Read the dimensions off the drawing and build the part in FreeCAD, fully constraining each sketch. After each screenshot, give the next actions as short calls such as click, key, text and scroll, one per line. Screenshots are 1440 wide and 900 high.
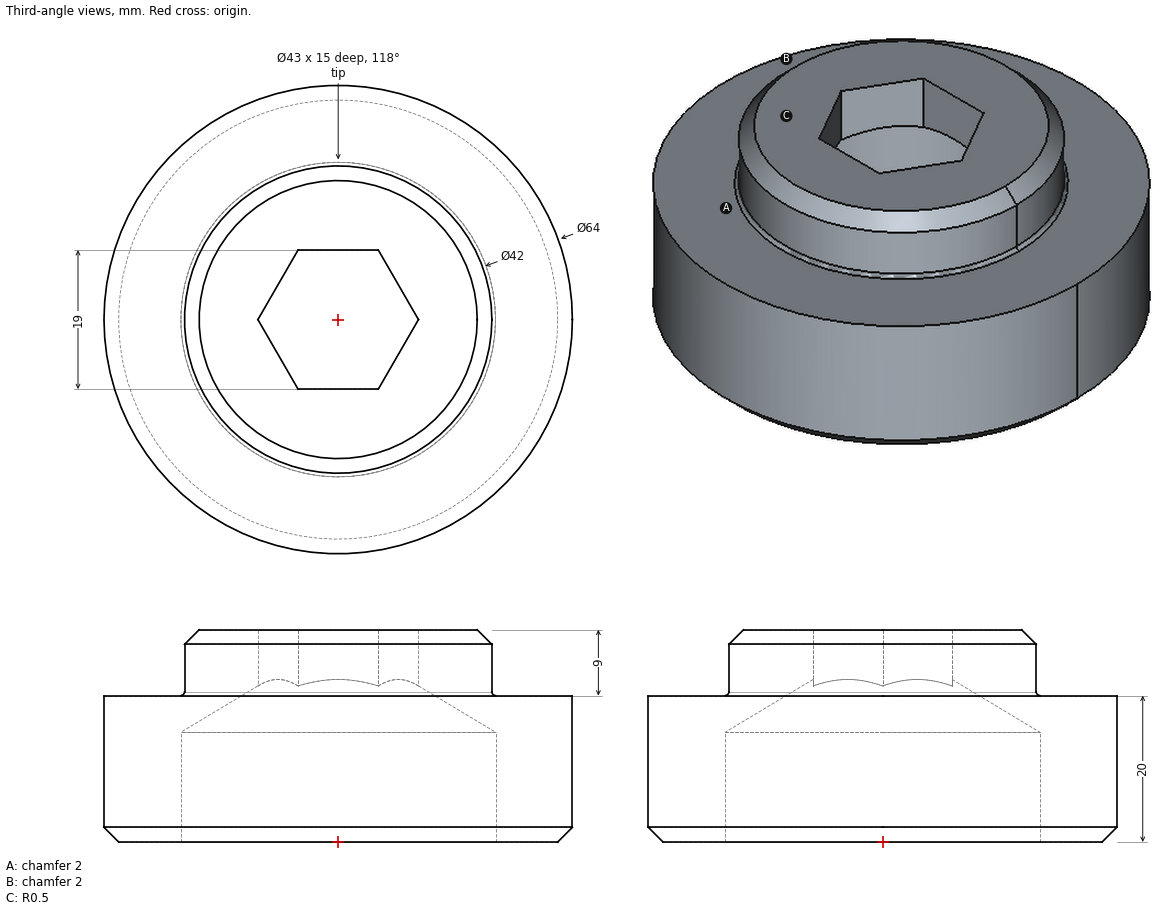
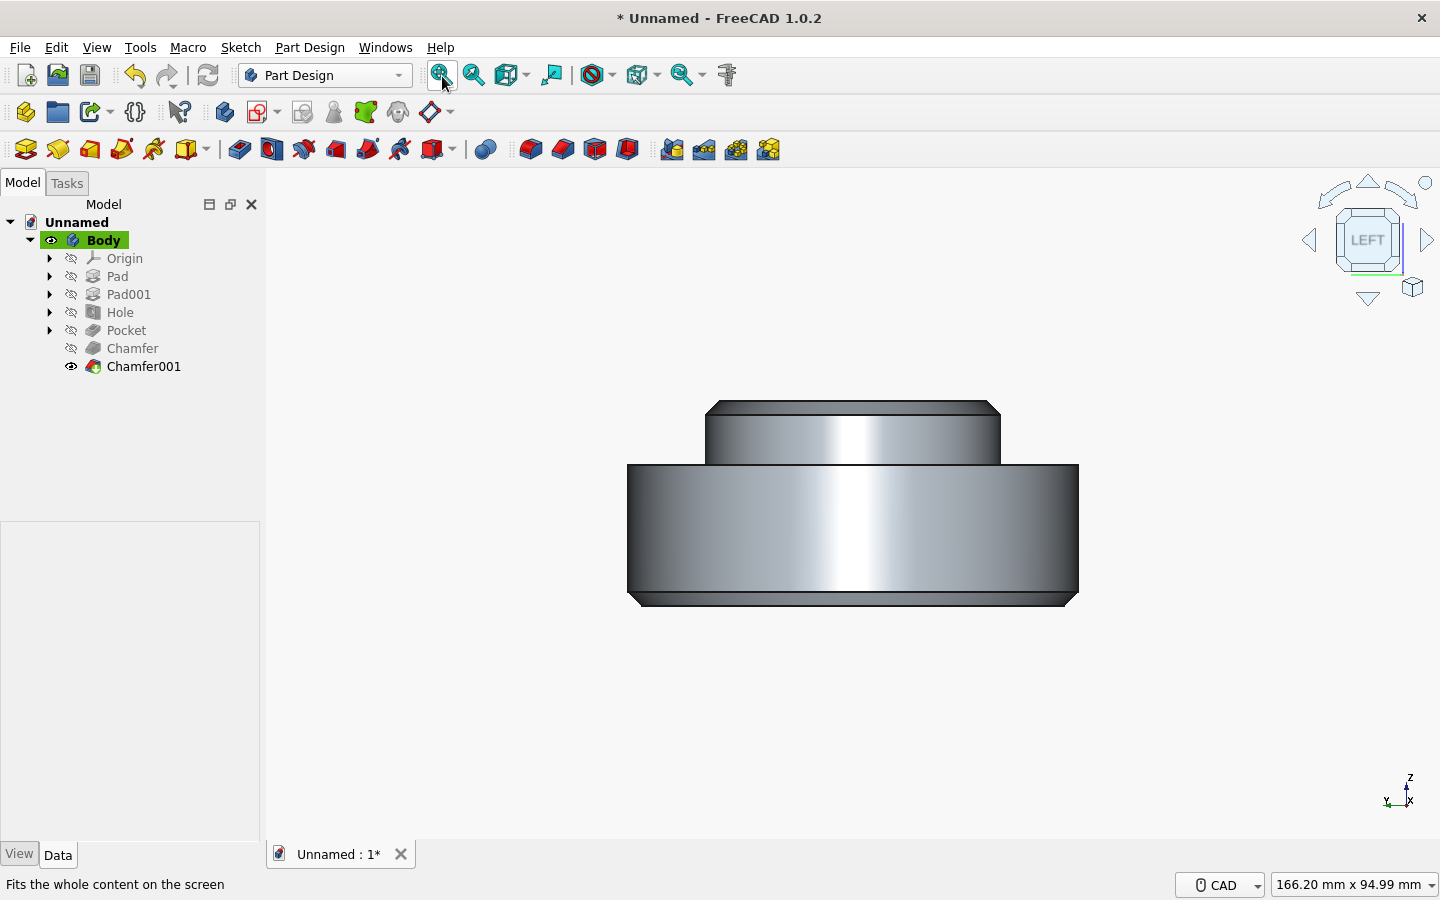
key(v)
key(3)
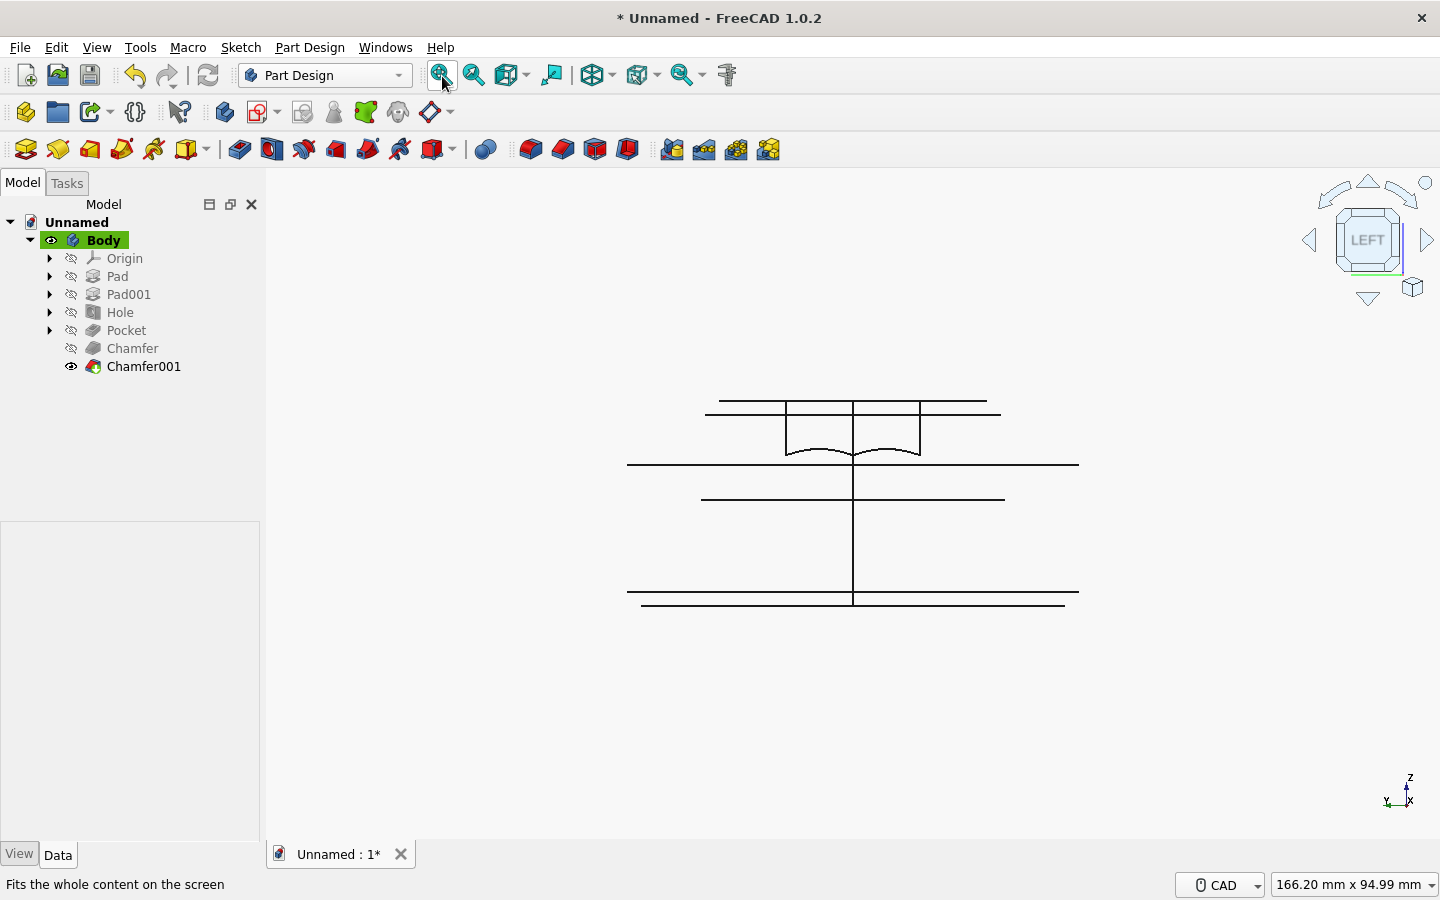
key(0)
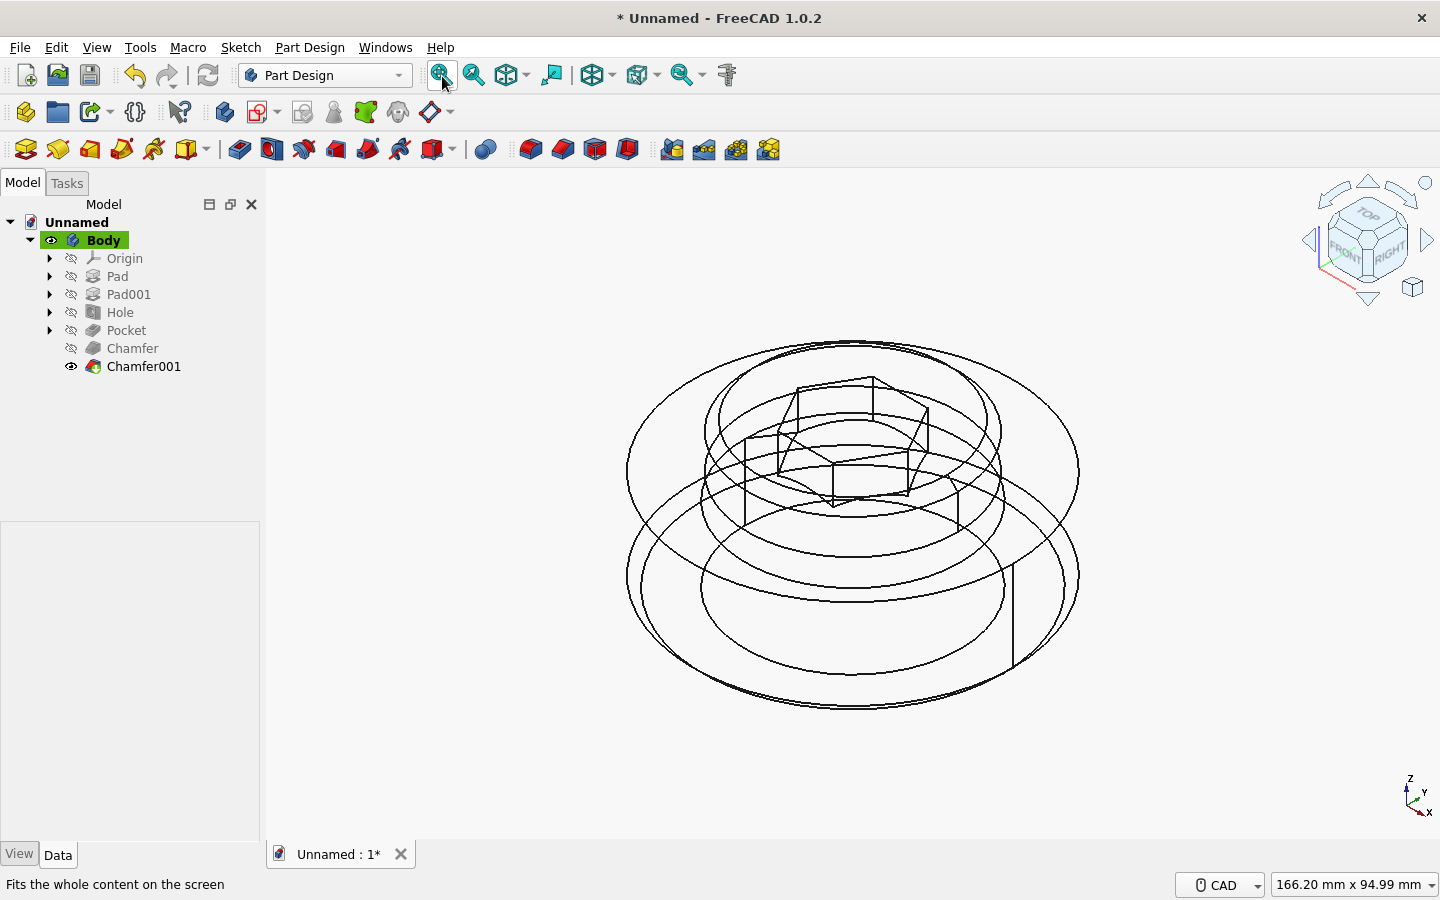
click(748, 410)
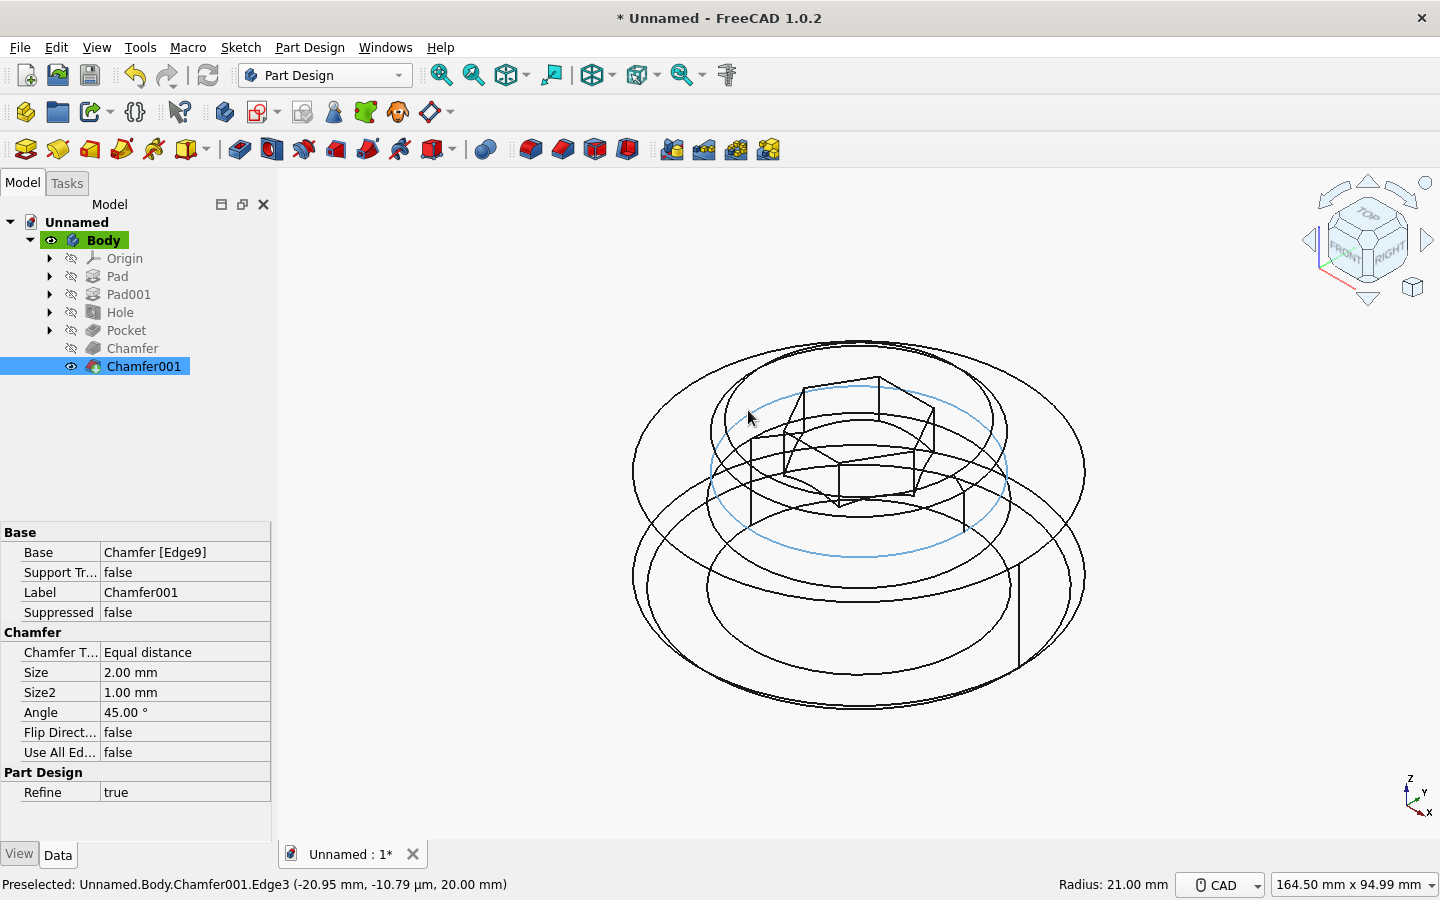
key(v)
key(1)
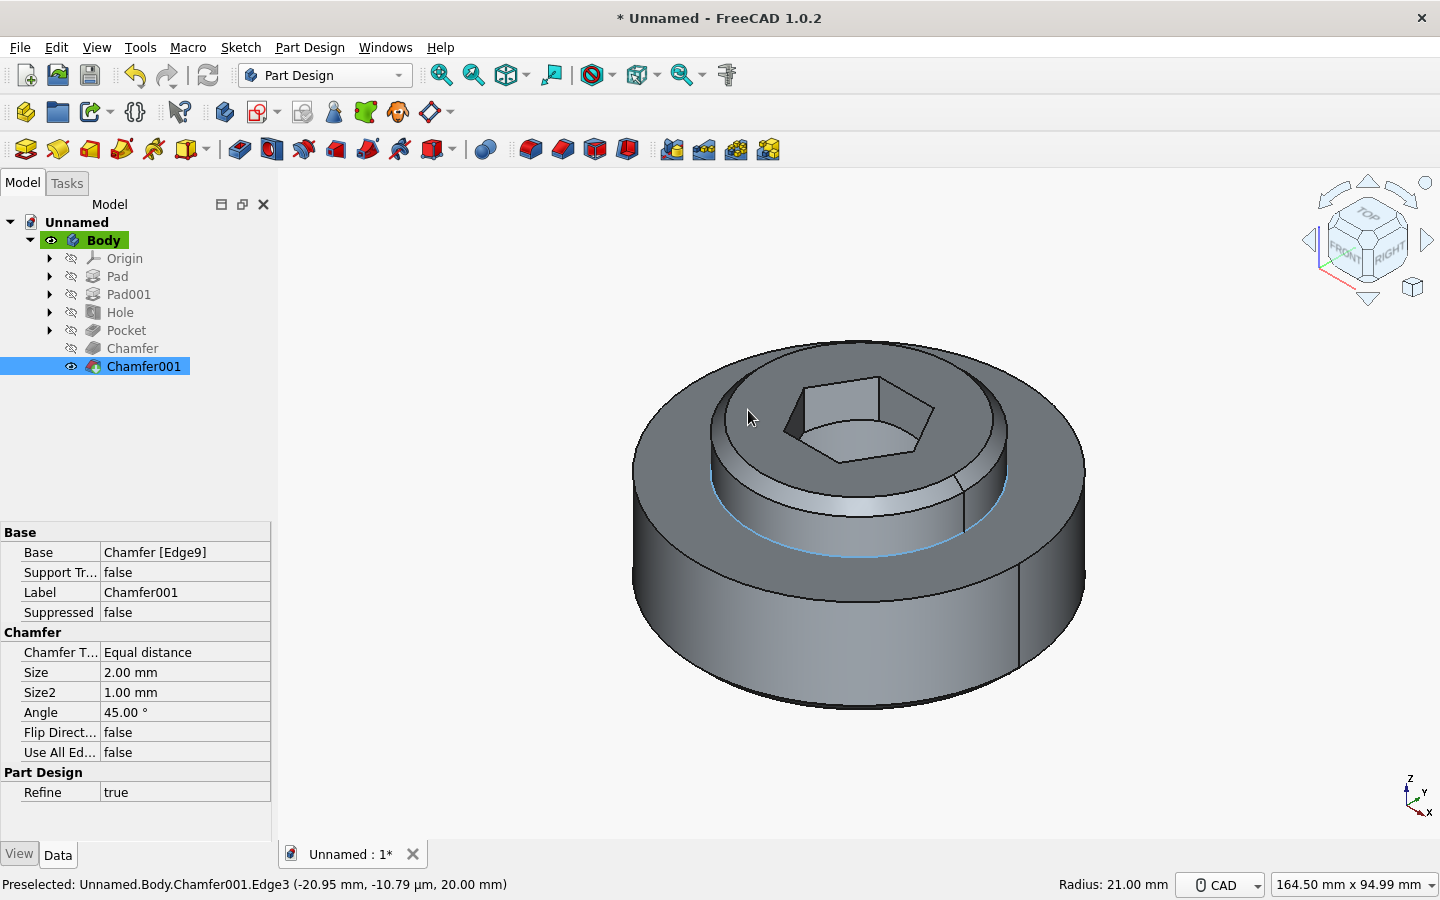
click(532, 150)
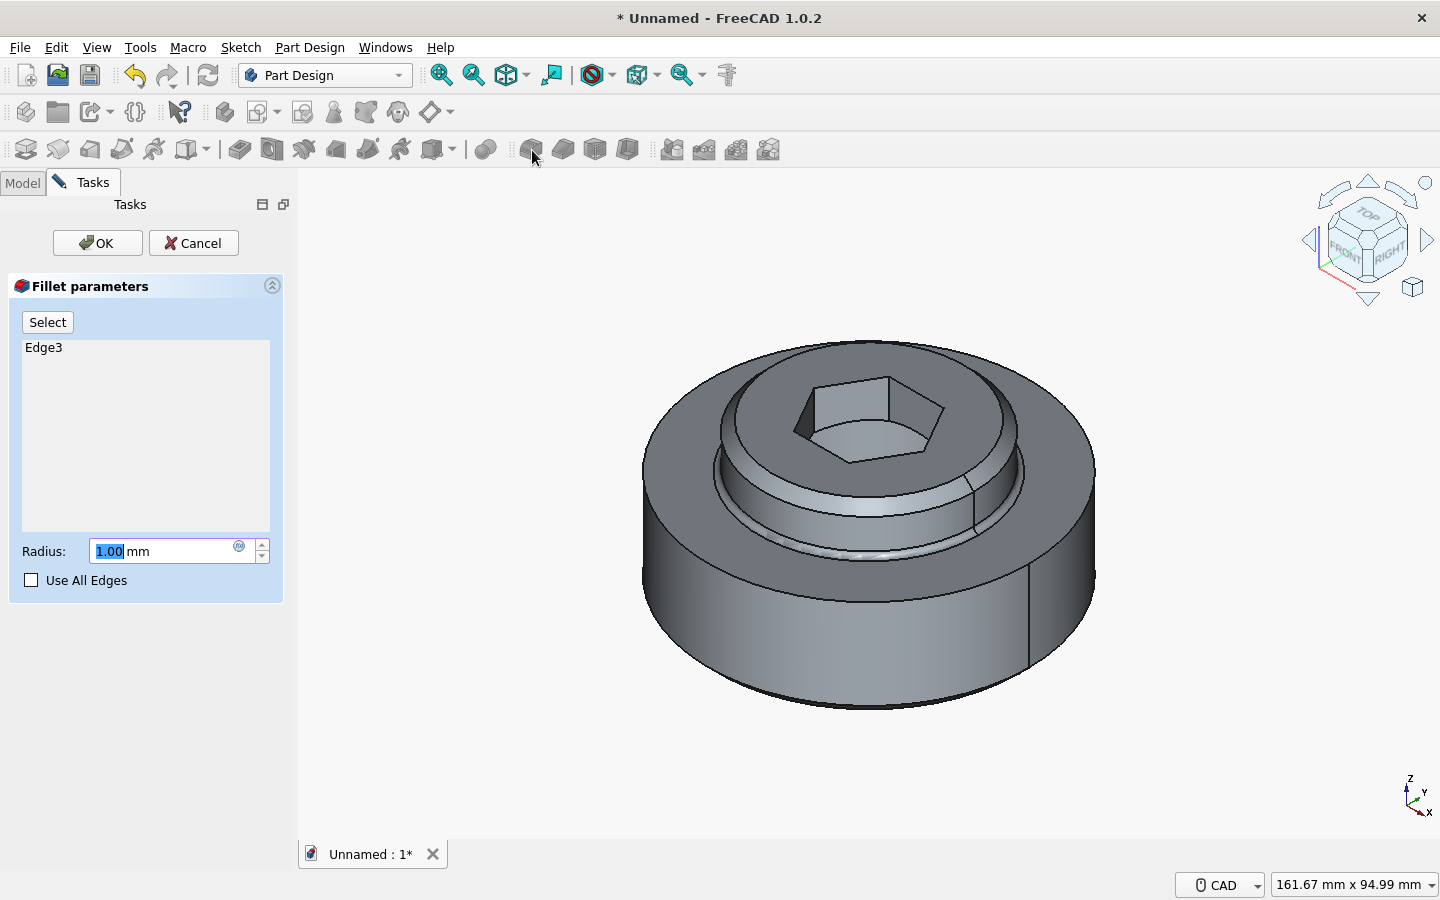
text(0.5)
key(Tab)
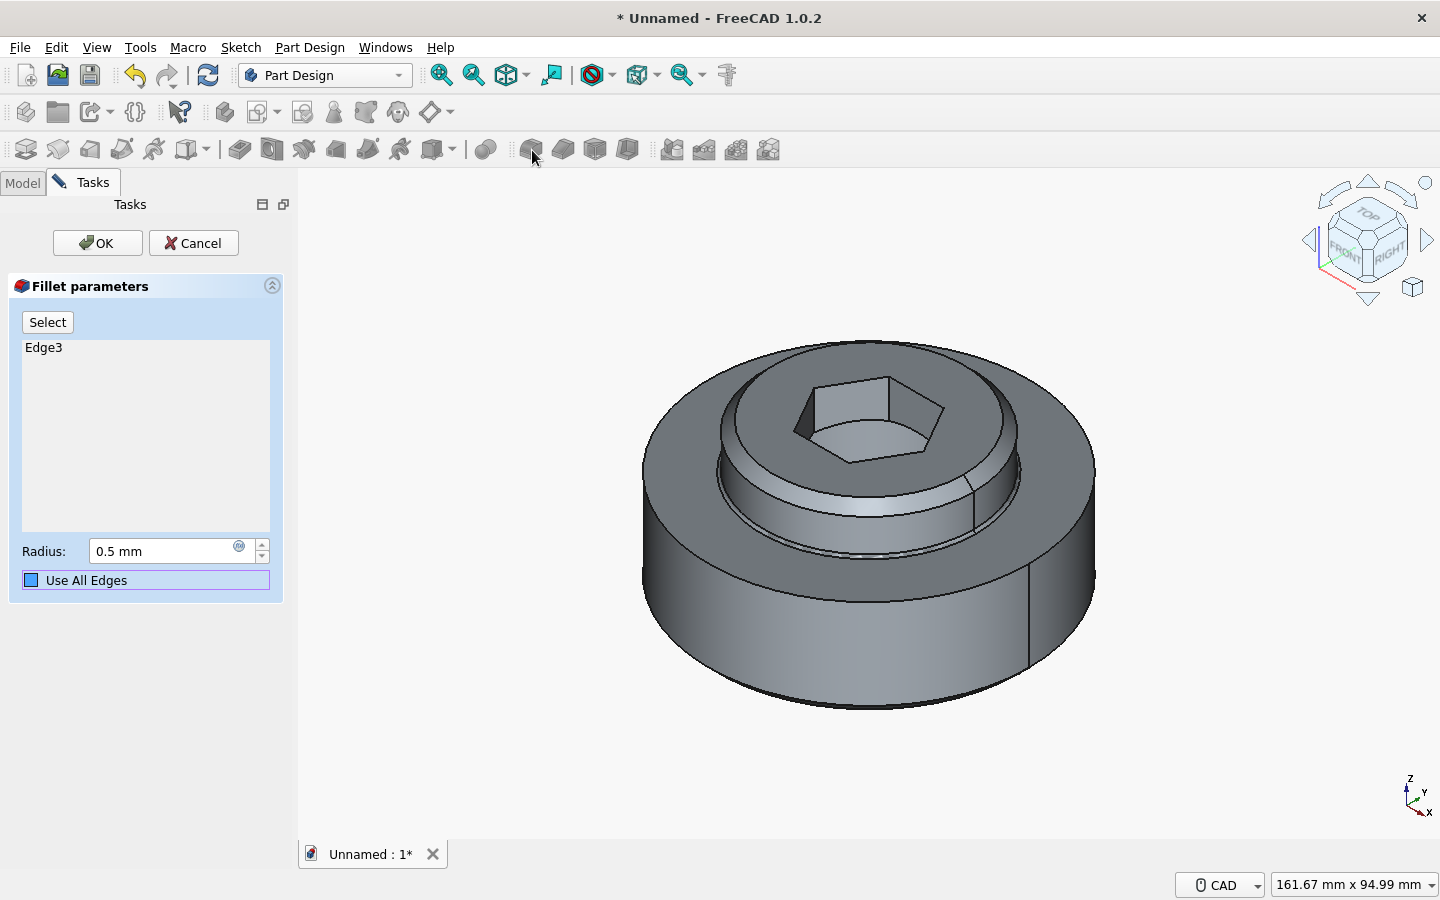
click(98, 243)